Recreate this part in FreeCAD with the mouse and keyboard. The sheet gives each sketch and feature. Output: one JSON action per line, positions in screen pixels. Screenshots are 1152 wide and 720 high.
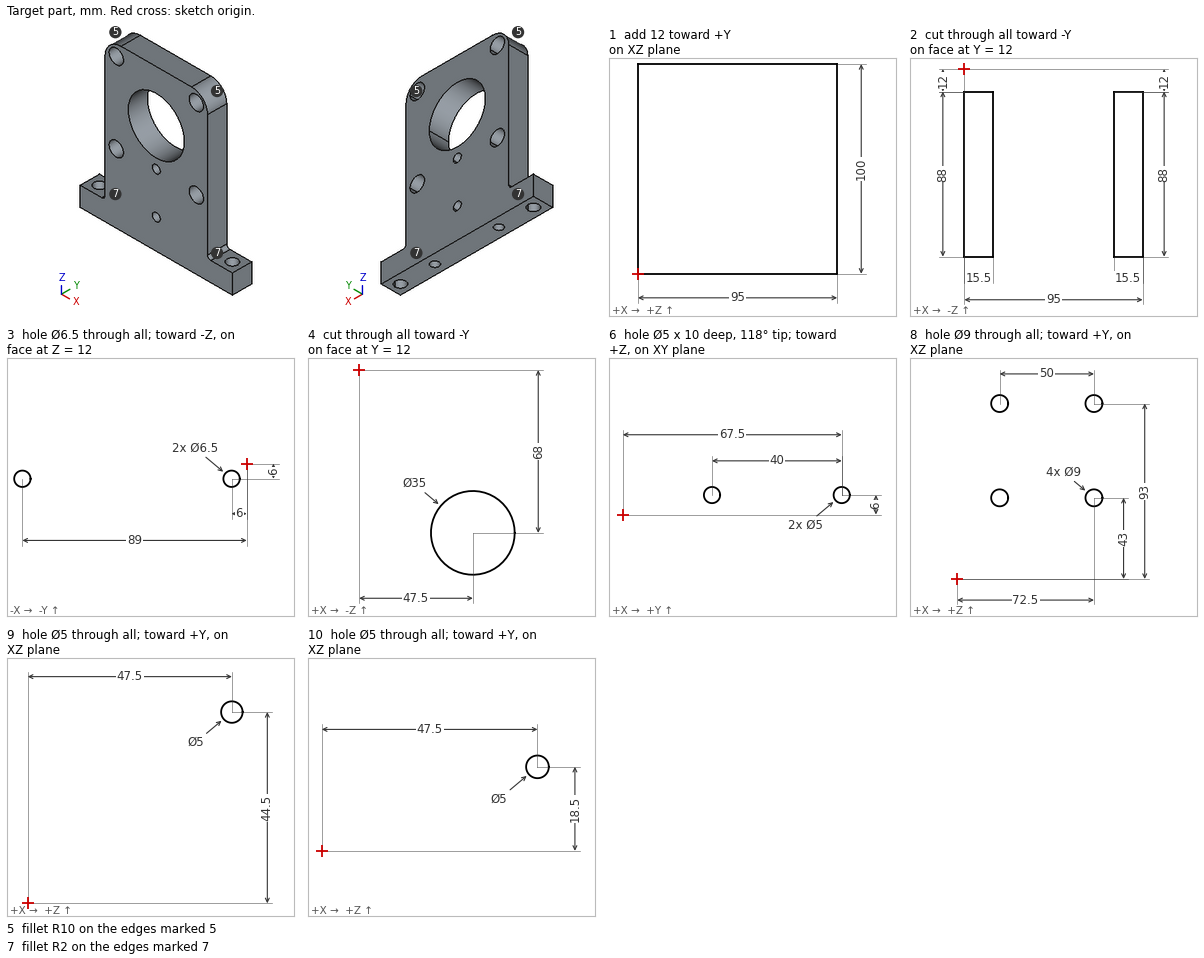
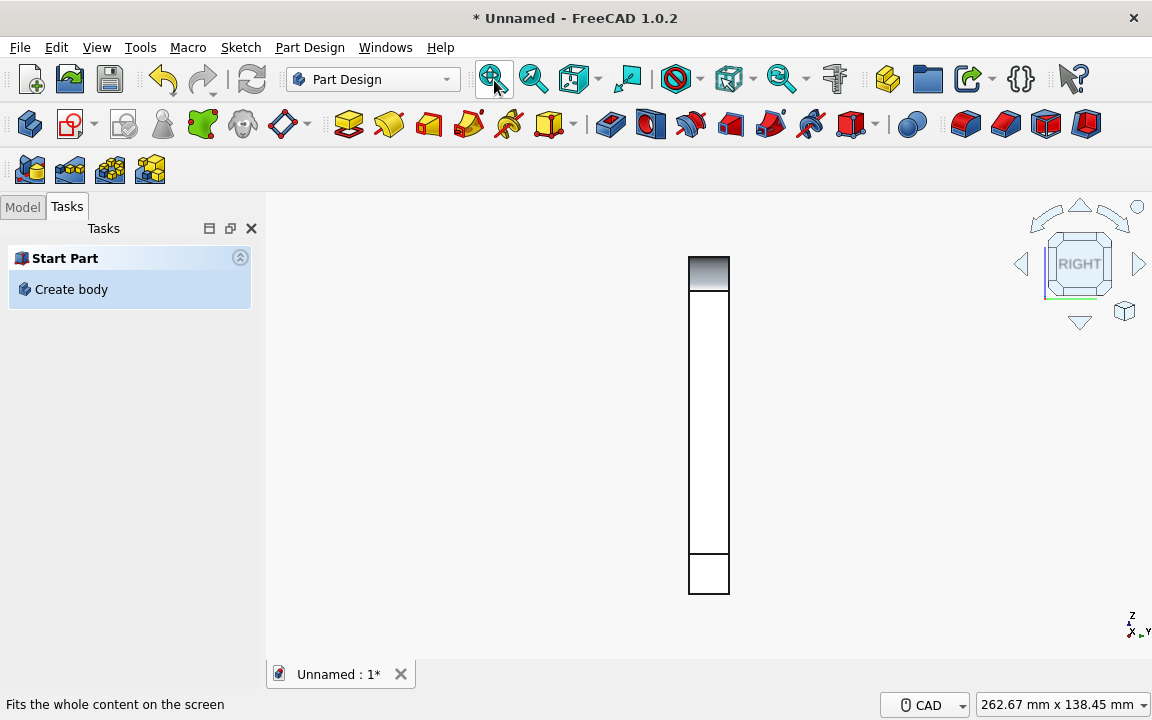
{"action": "key", "text": "5"}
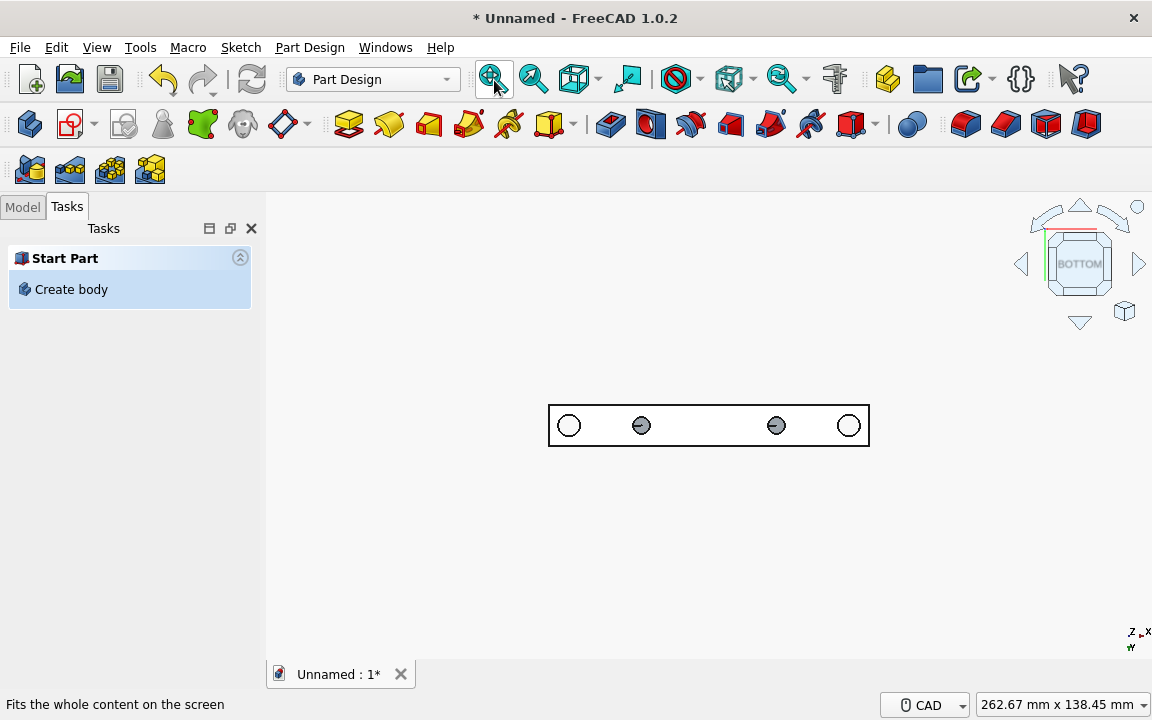
{"action": "left_click", "coordinate": [494, 80]}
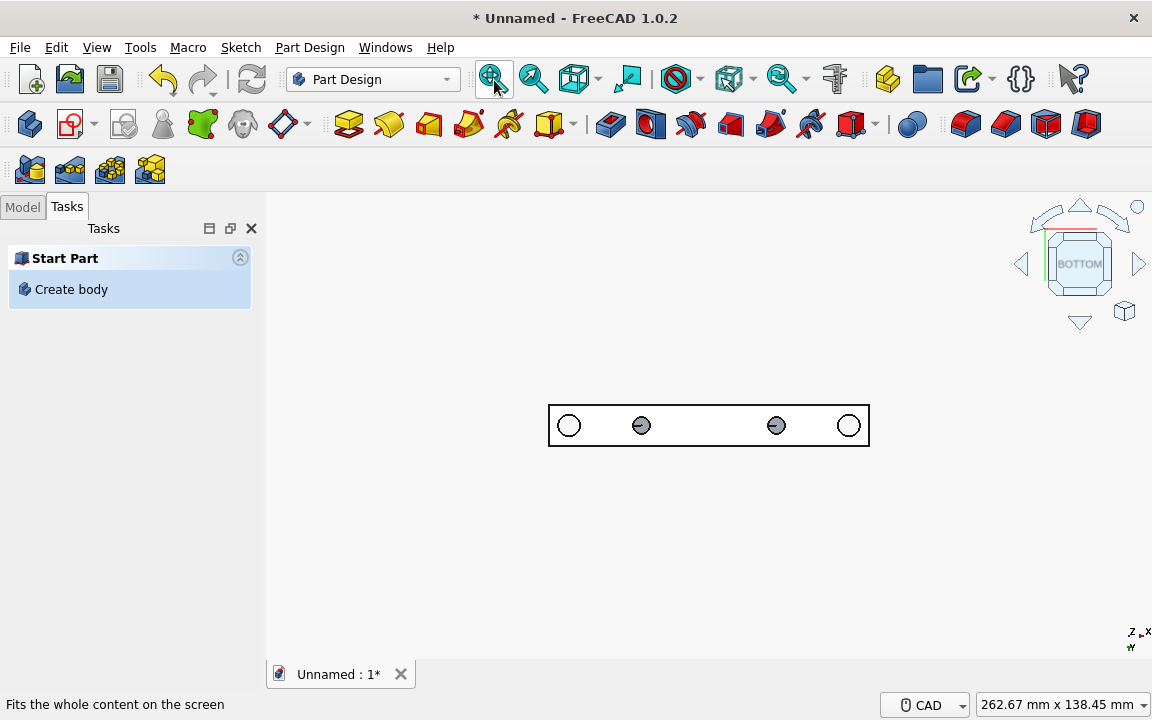
{"action": "key", "text": "4"}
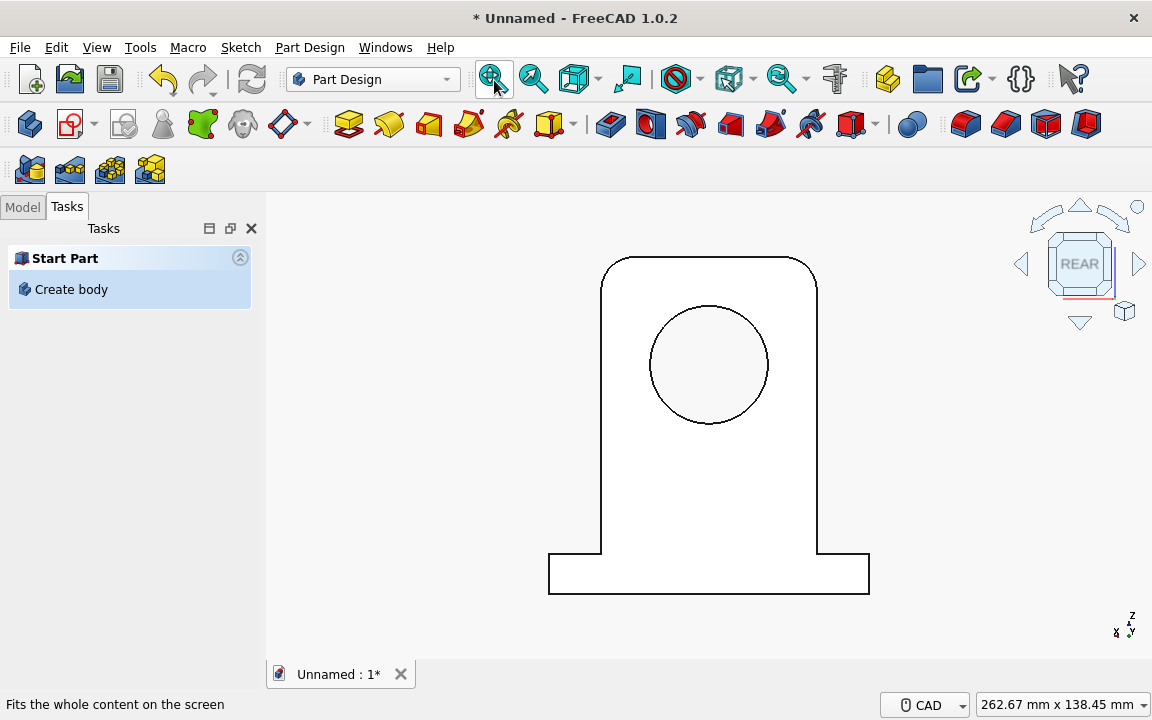
{"action": "key", "text": "6"}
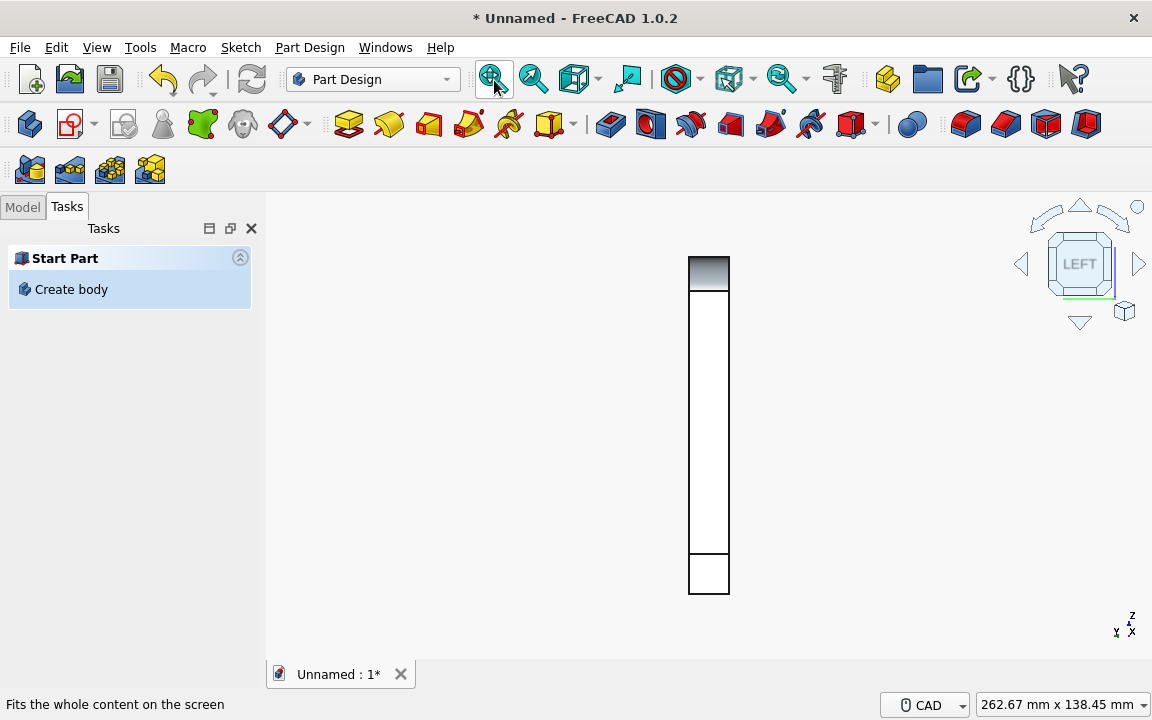
{"action": "key", "text": "v 3"}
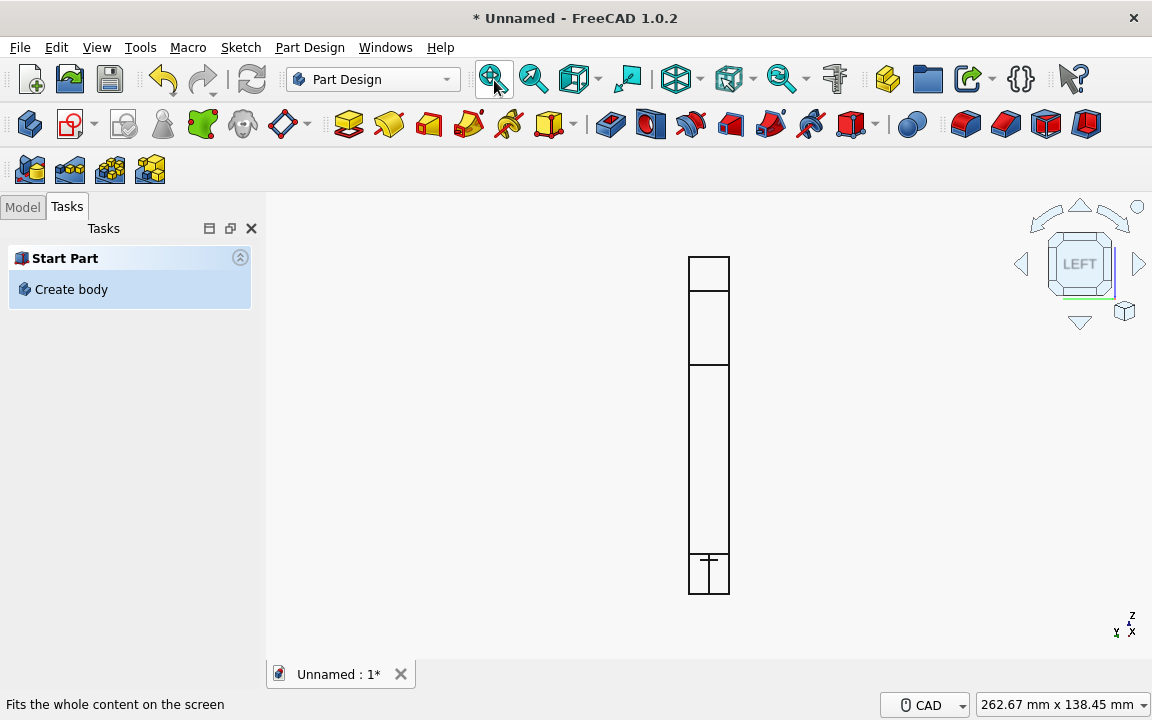
{"action": "key", "text": "0"}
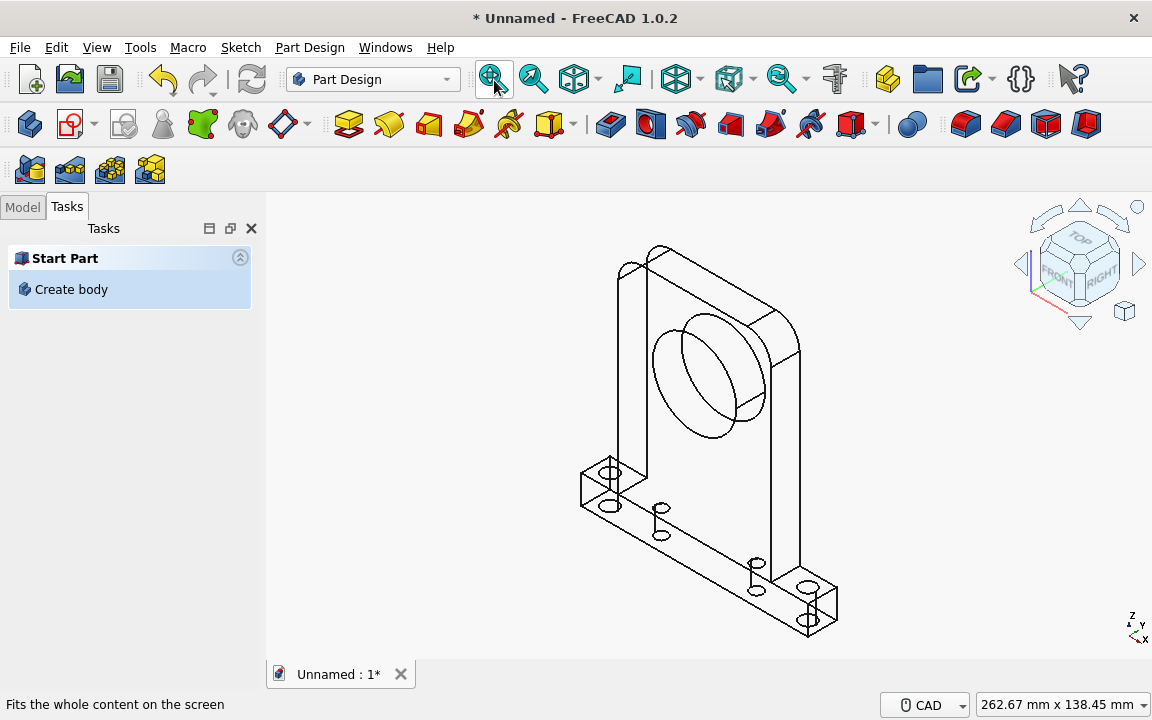
{"action": "left_click", "coordinate": [633, 485]}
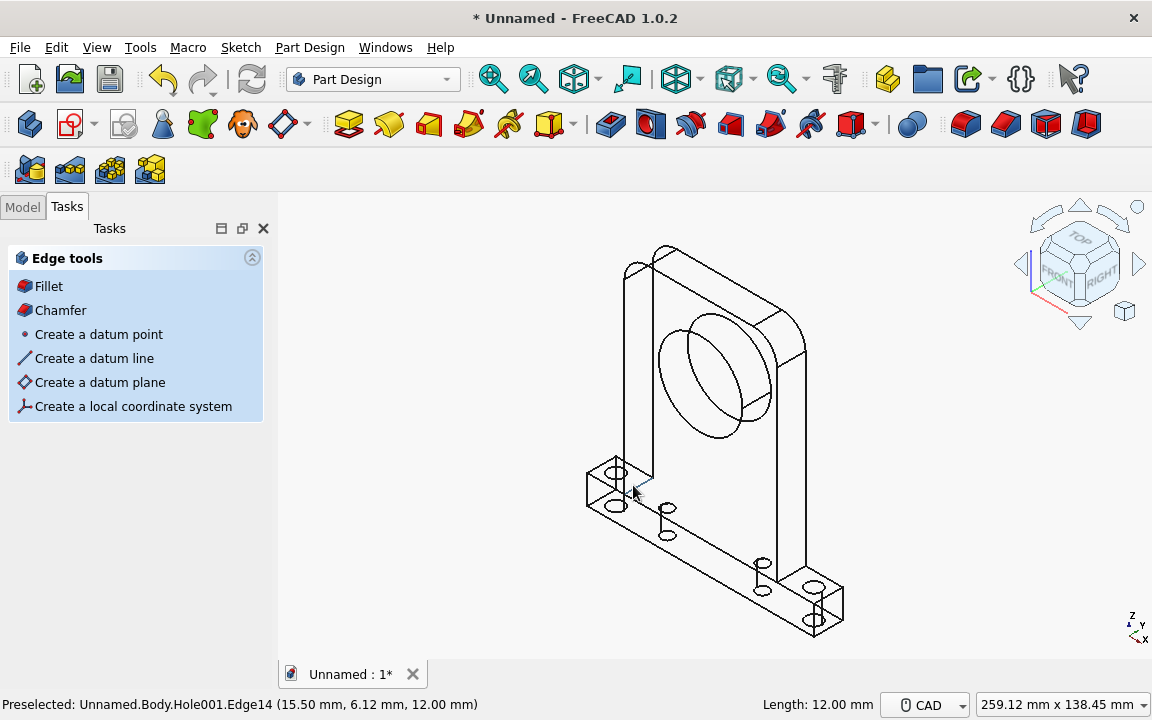
{"action": "left_click", "coordinate": [791, 573], "text": "ctrl"}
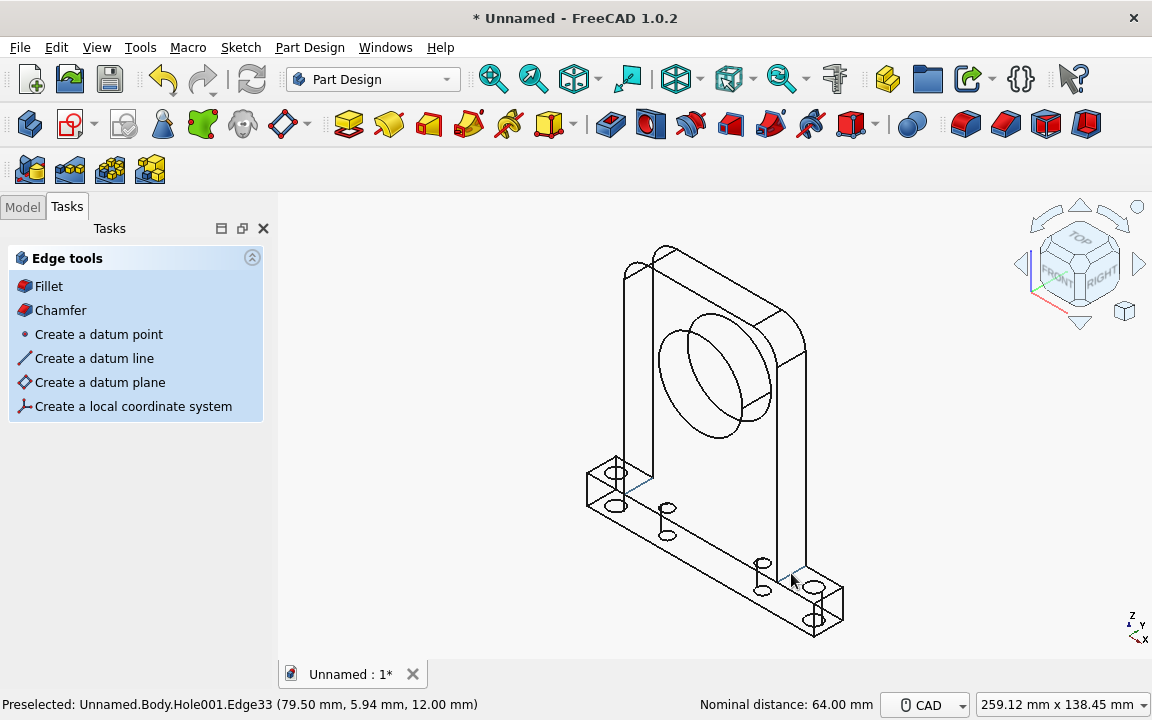
{"action": "key", "text": "v 1"}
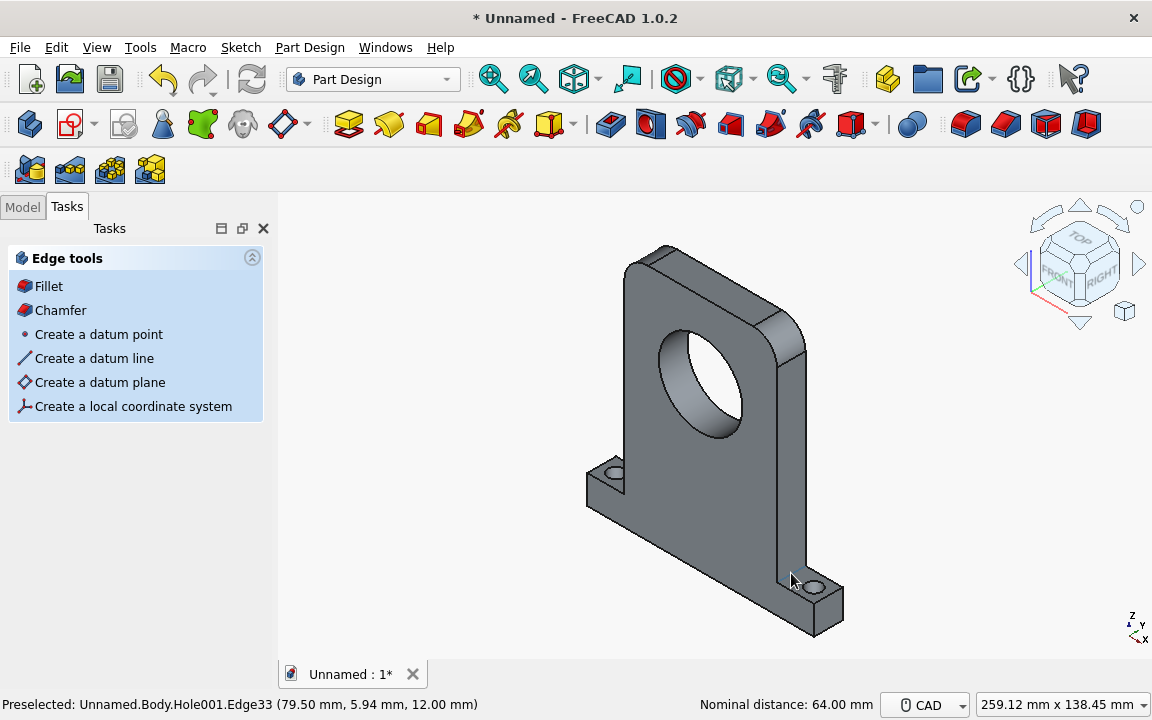
{"action": "left_click", "coordinate": [966, 124]}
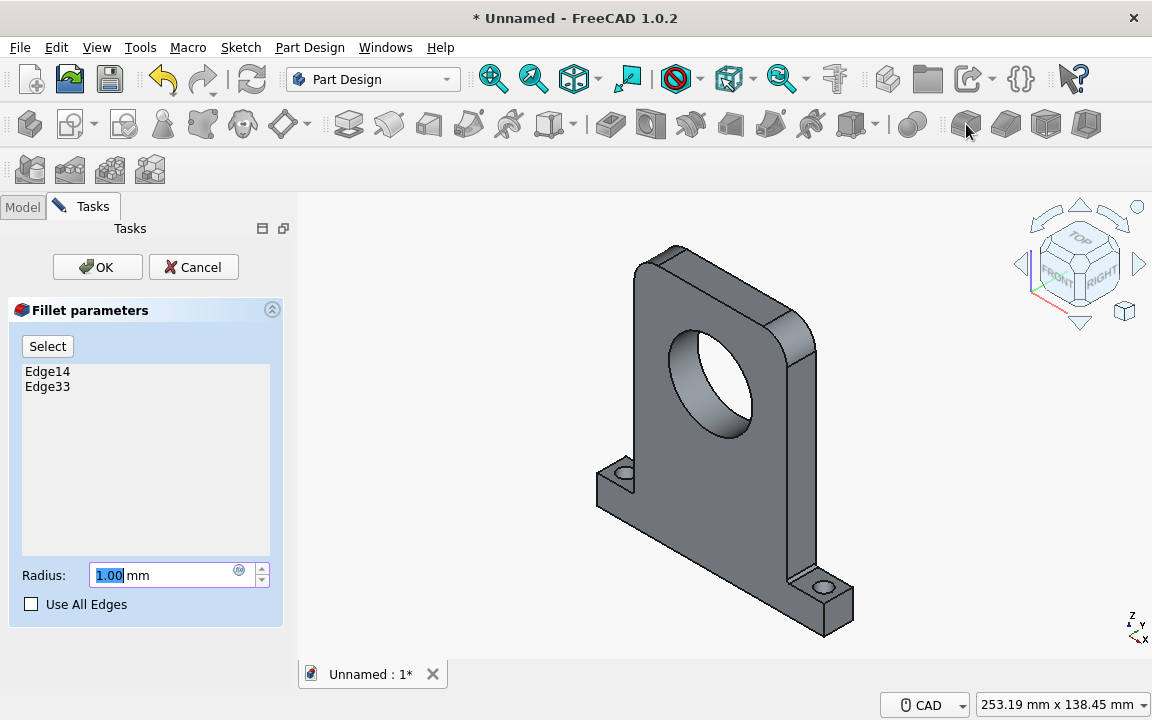
{"action": "type", "text": "2"}
{"action": "key", "text": "Tab"}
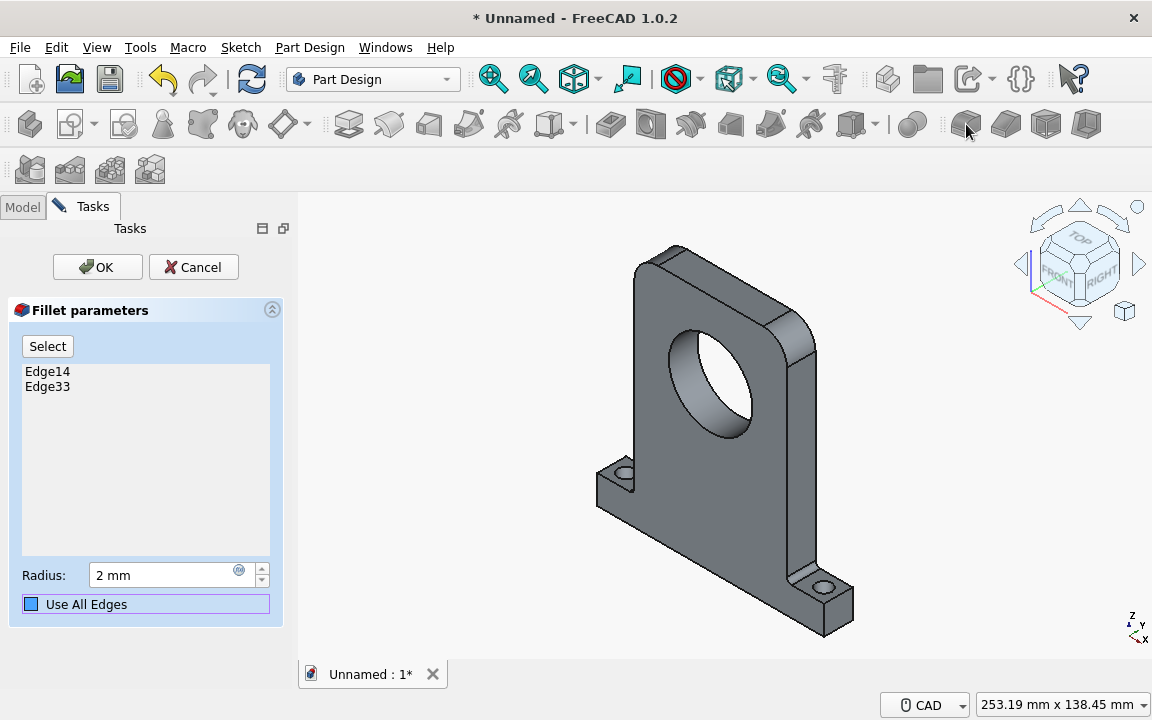
{"action": "left_click", "coordinate": [98, 267]}